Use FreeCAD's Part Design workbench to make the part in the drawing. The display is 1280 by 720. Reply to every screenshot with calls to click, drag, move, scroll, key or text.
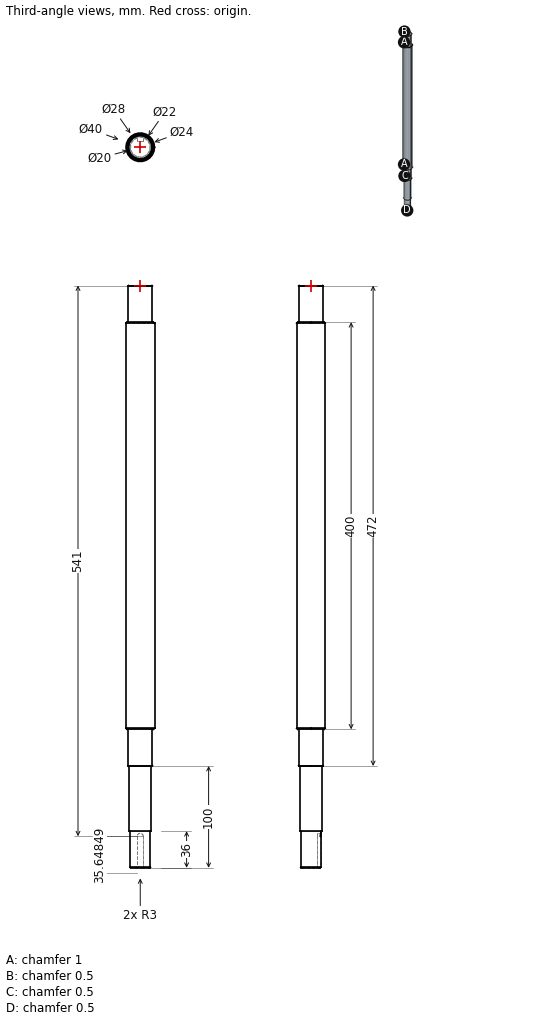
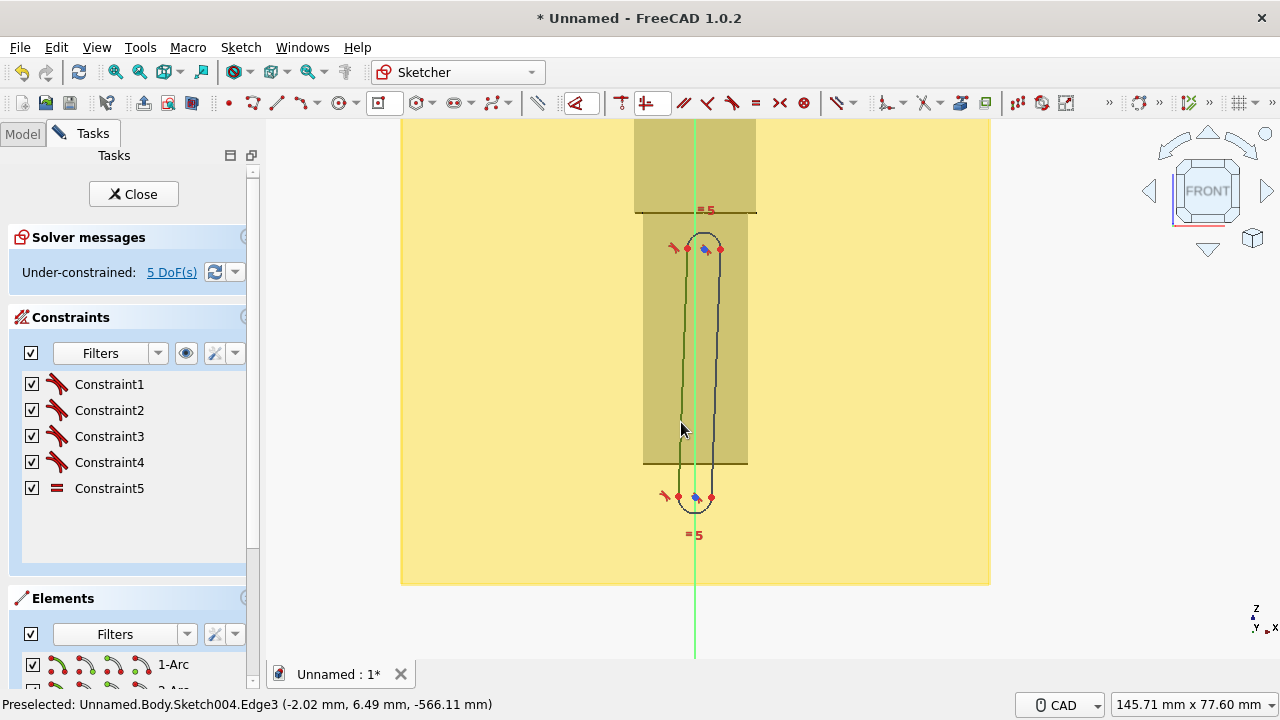
click(666, 104)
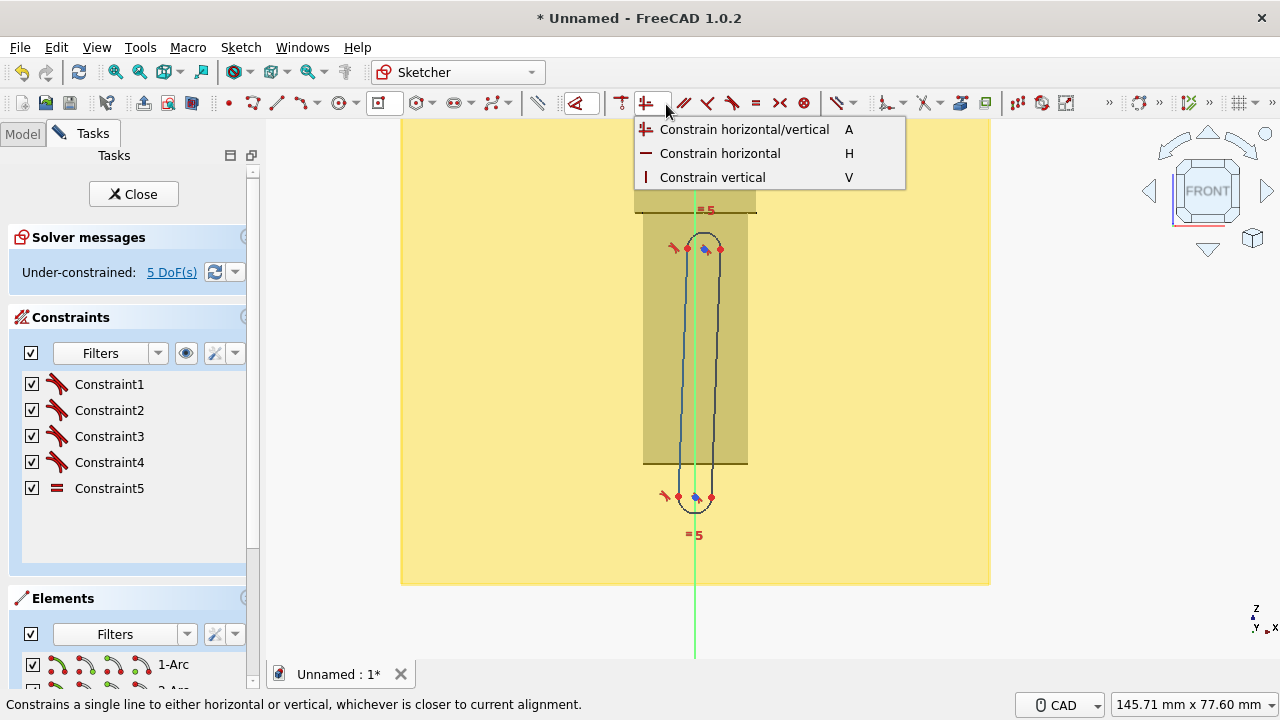
click(770, 177)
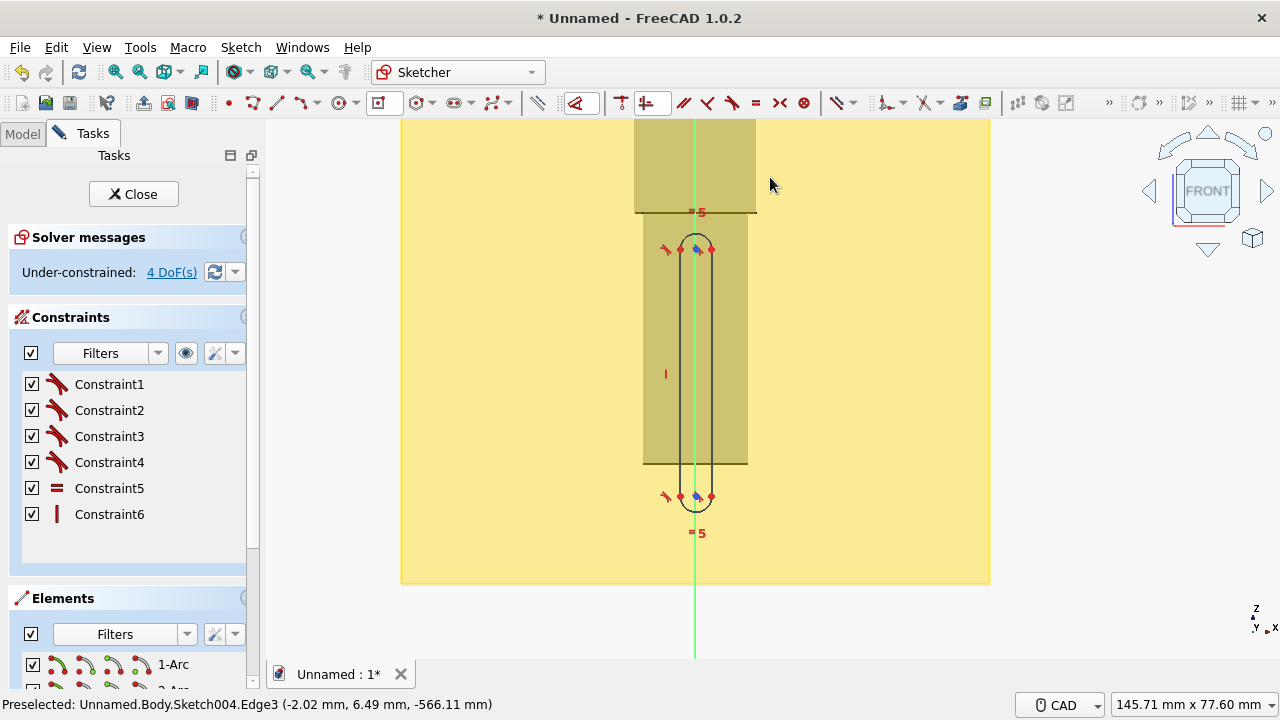
click(696, 496)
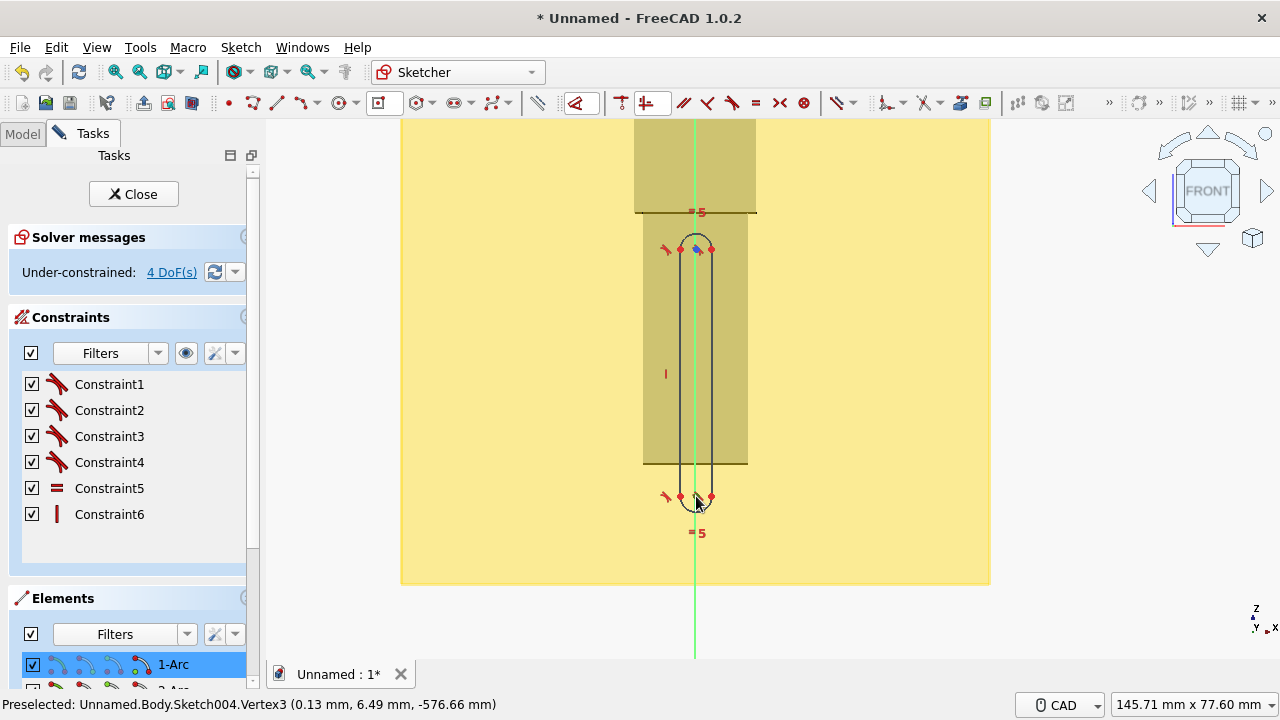
click(695, 596)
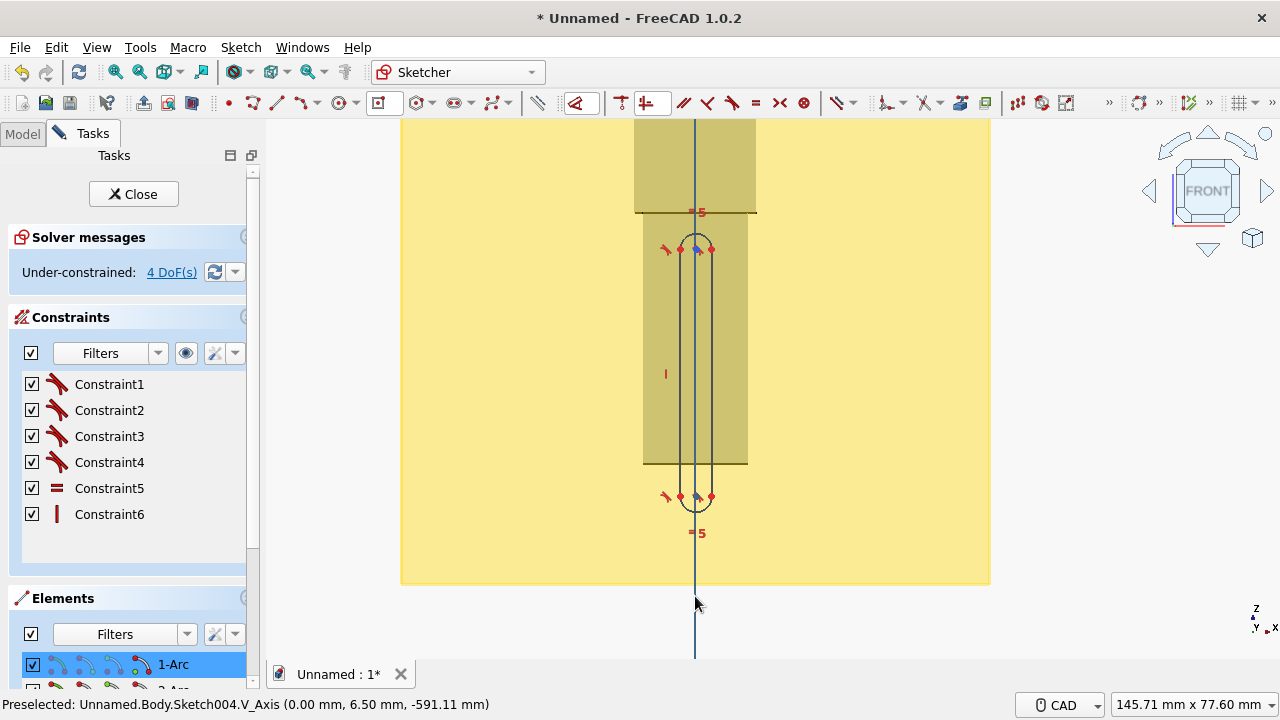
key(c)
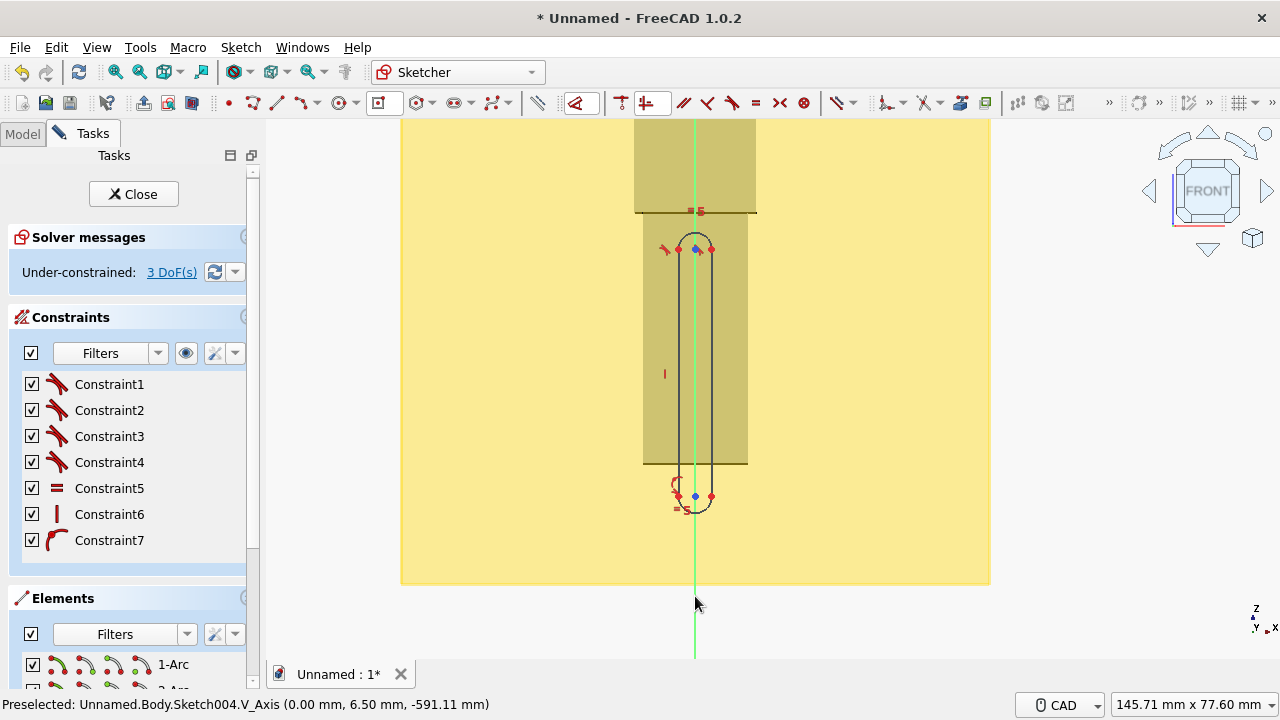
scroll(685, 510, up, 4)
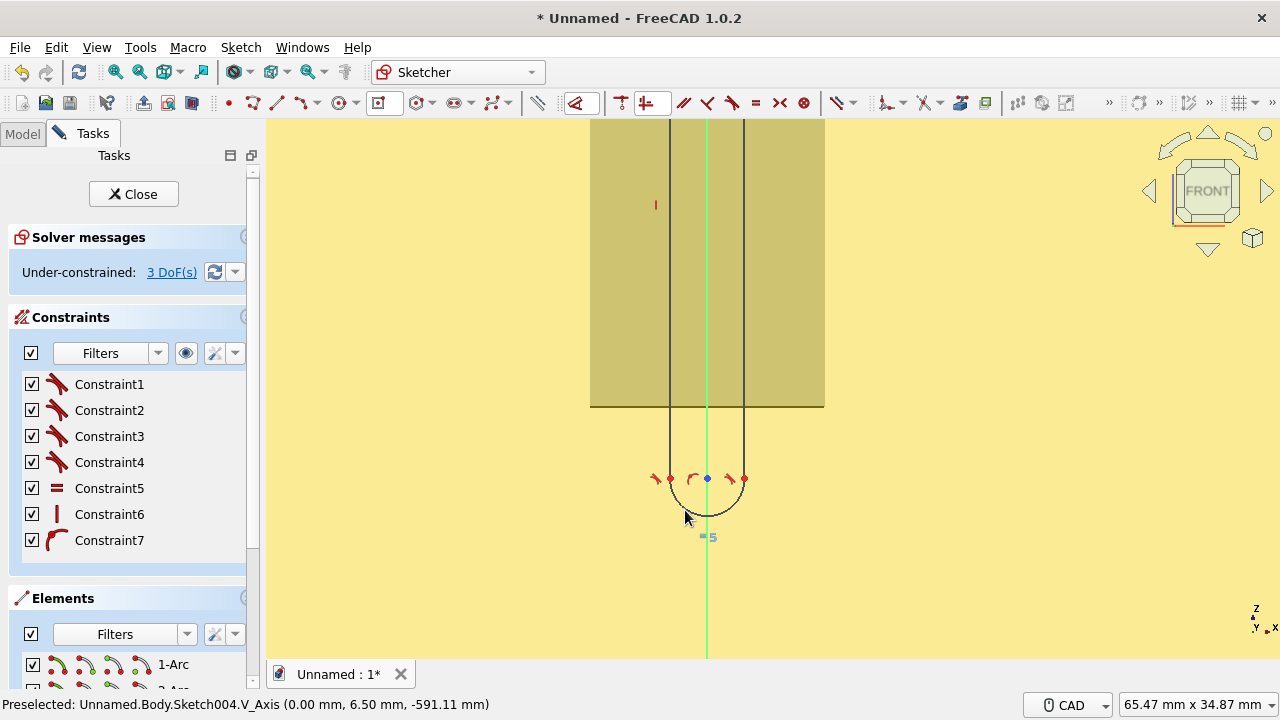
click(685, 509)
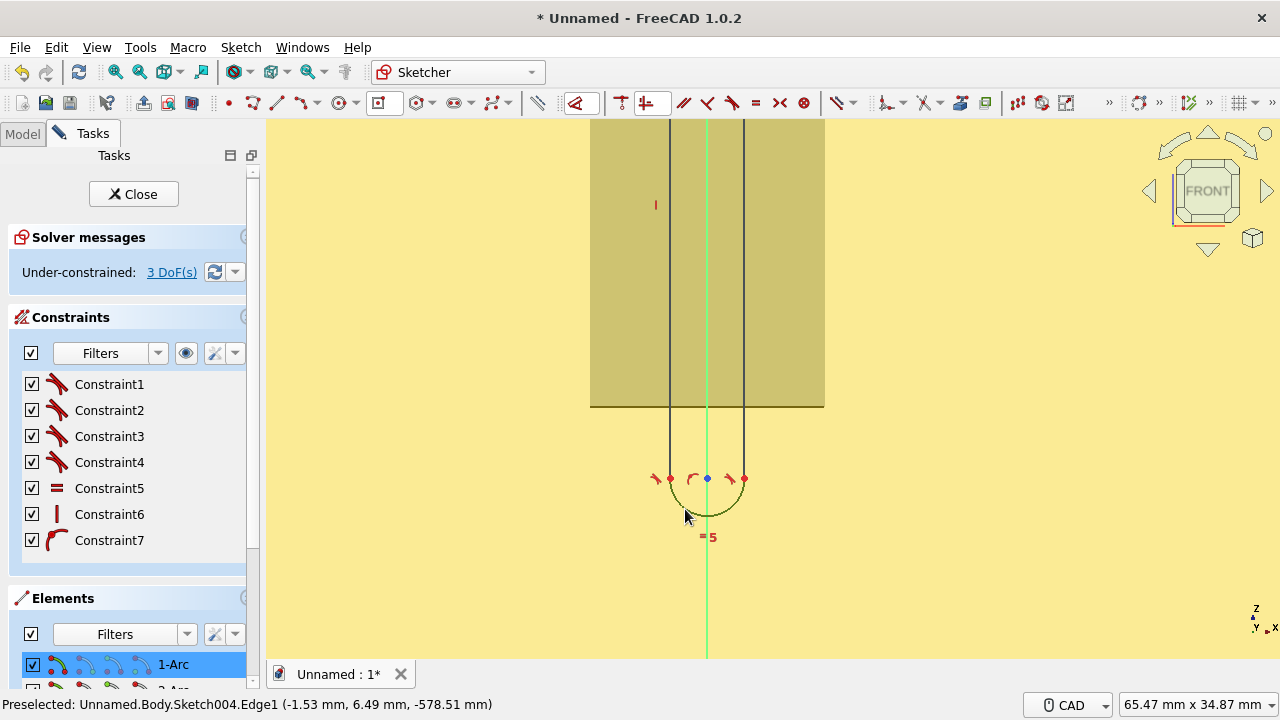
click(594, 104)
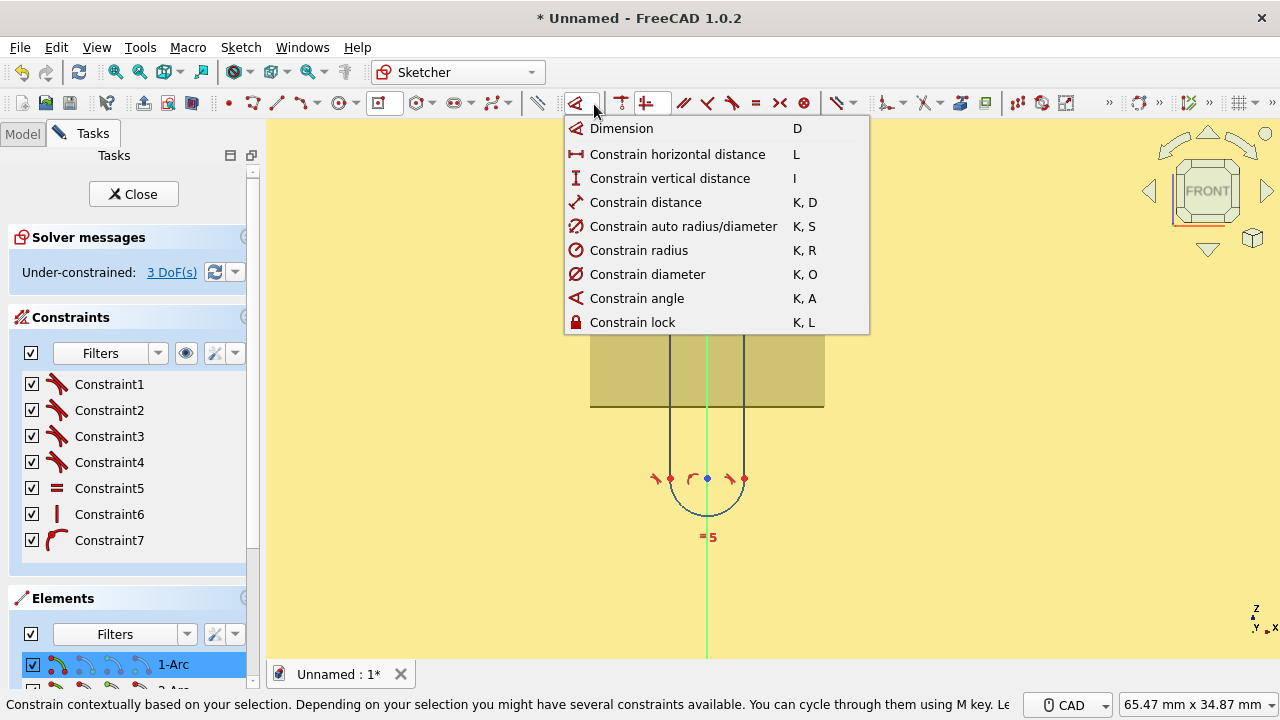
click(717, 250)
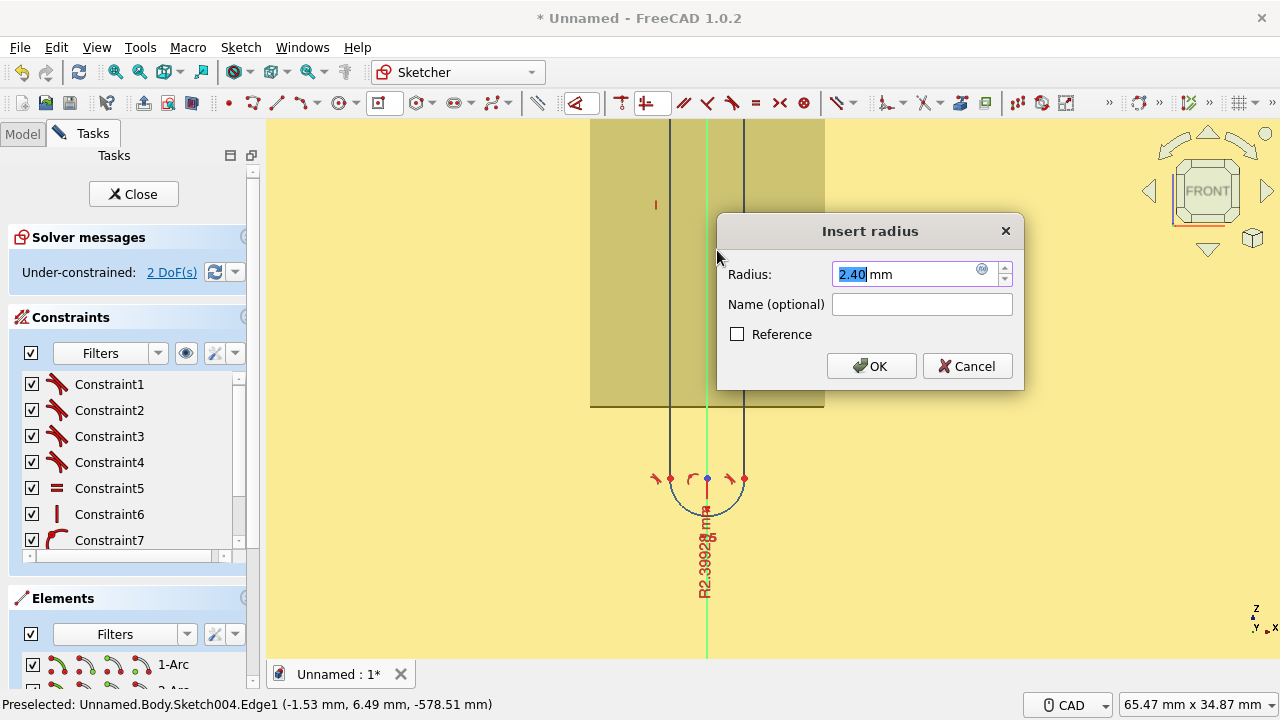
text(3)
key(Return)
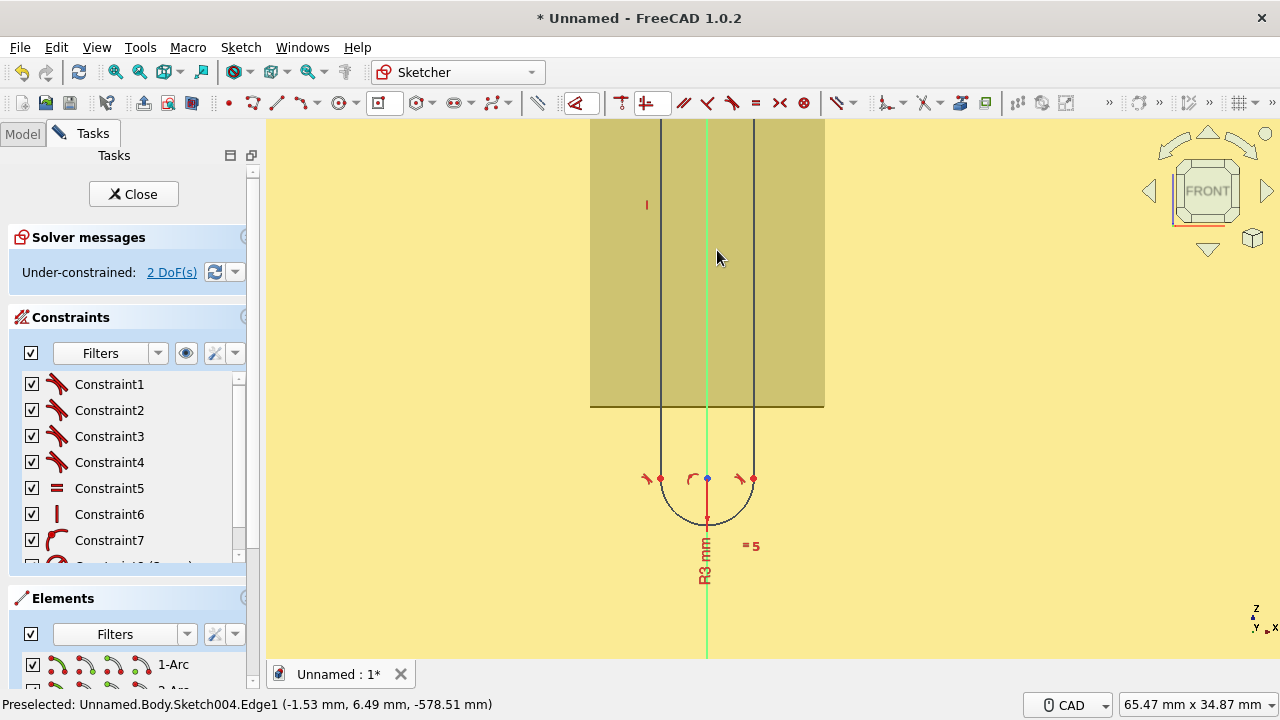
scroll(701, 616, down, 3)